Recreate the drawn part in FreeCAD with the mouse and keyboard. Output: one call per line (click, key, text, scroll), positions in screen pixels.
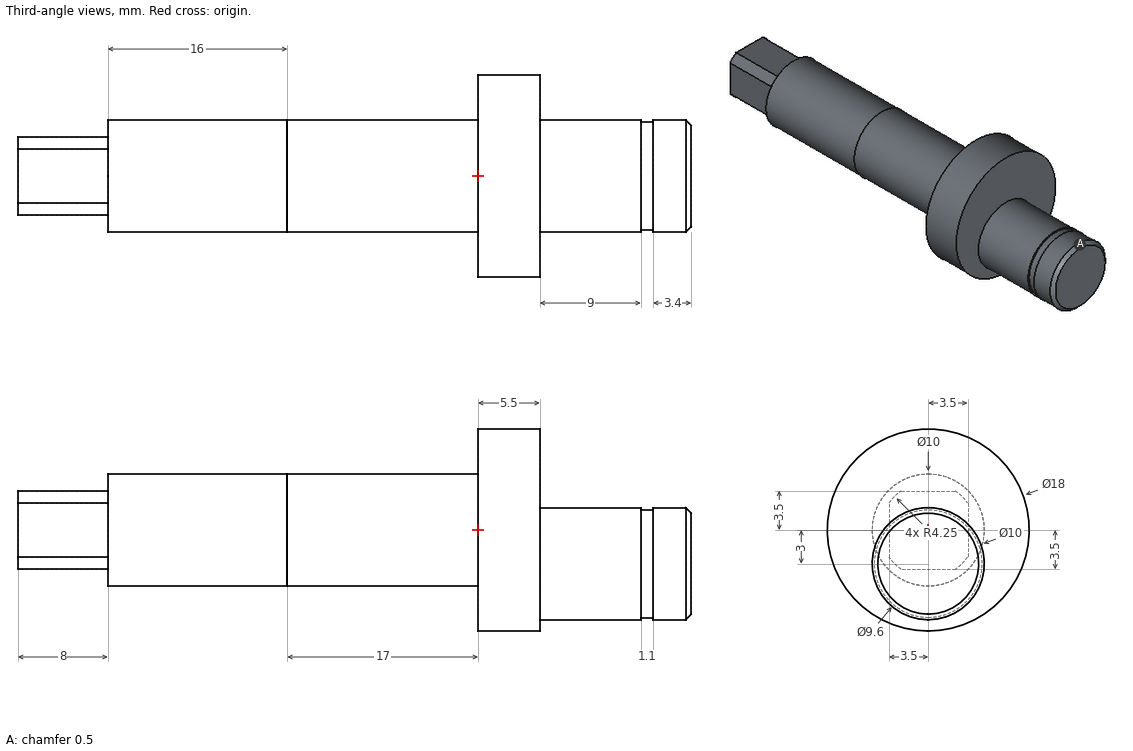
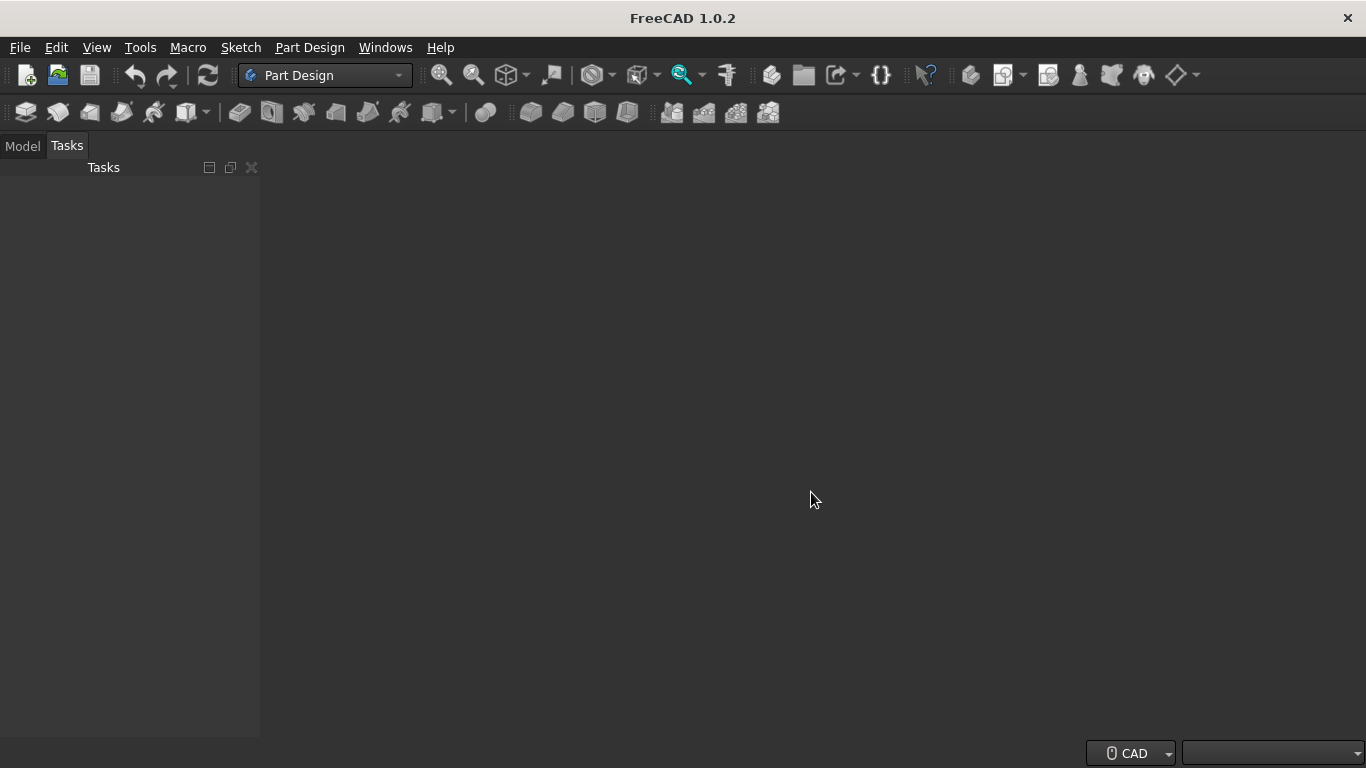
key(ctrl+n)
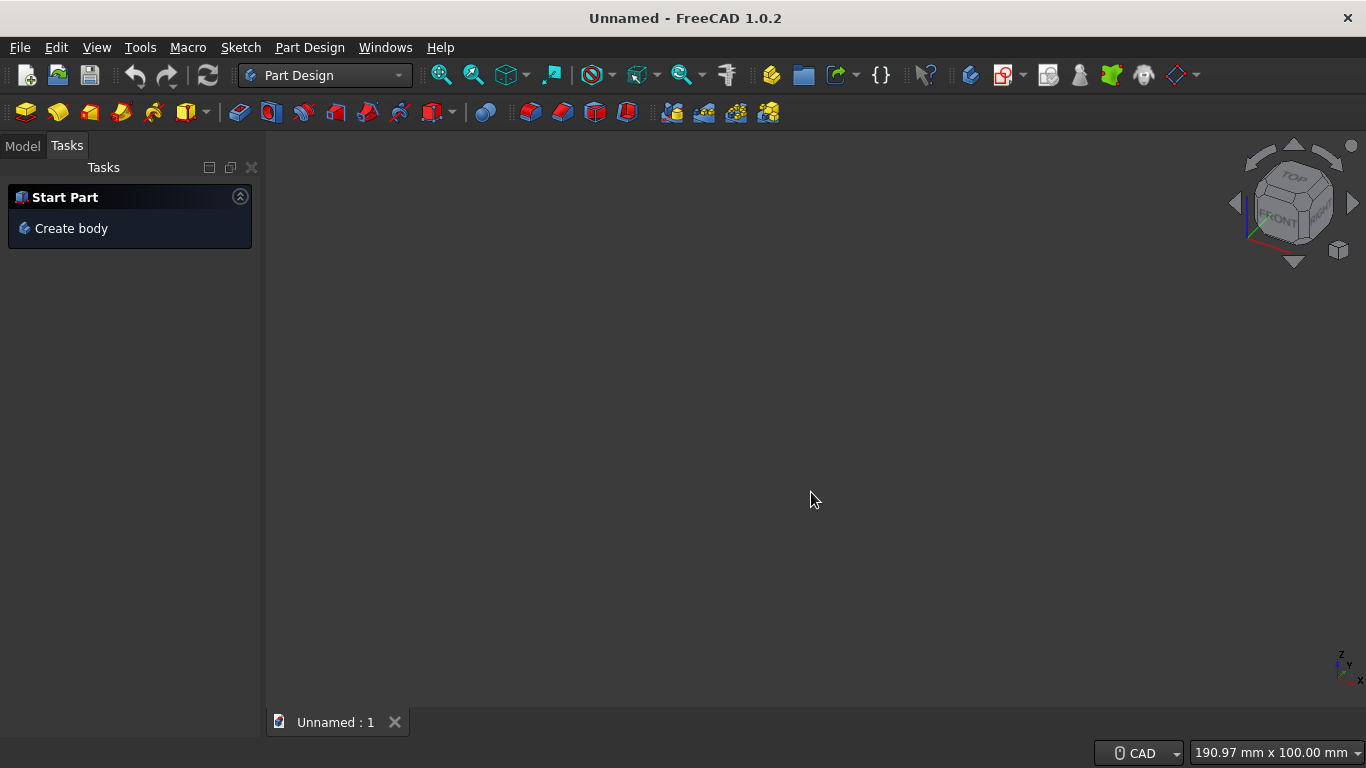
click(1004, 76)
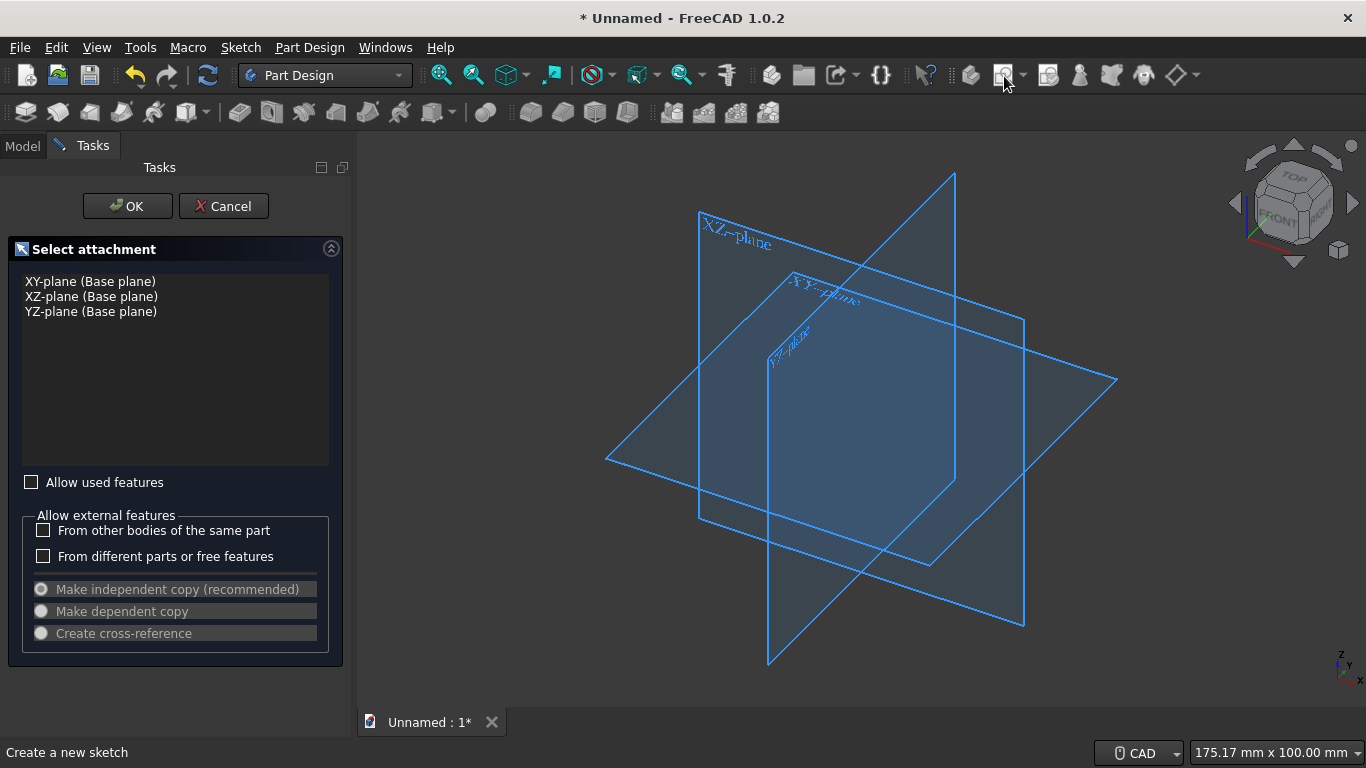
click(82, 312)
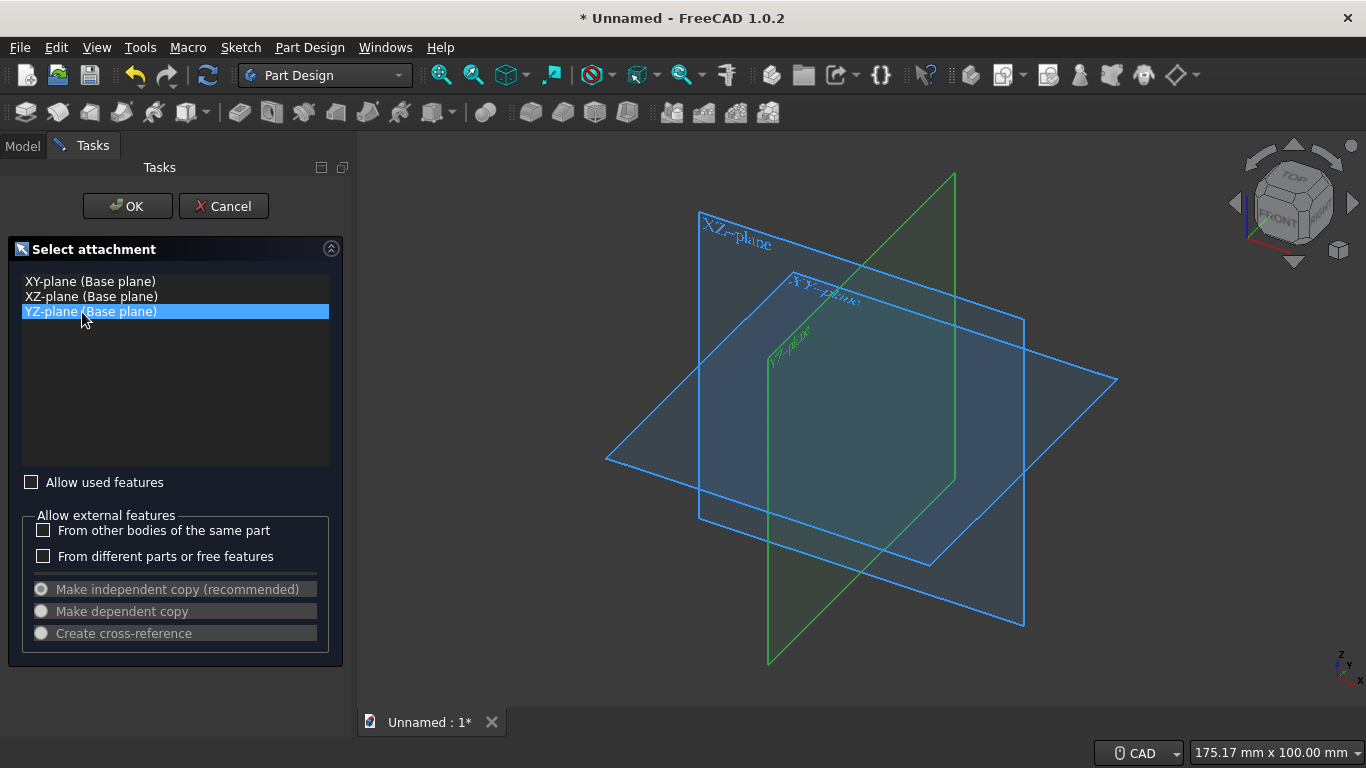
click(128, 206)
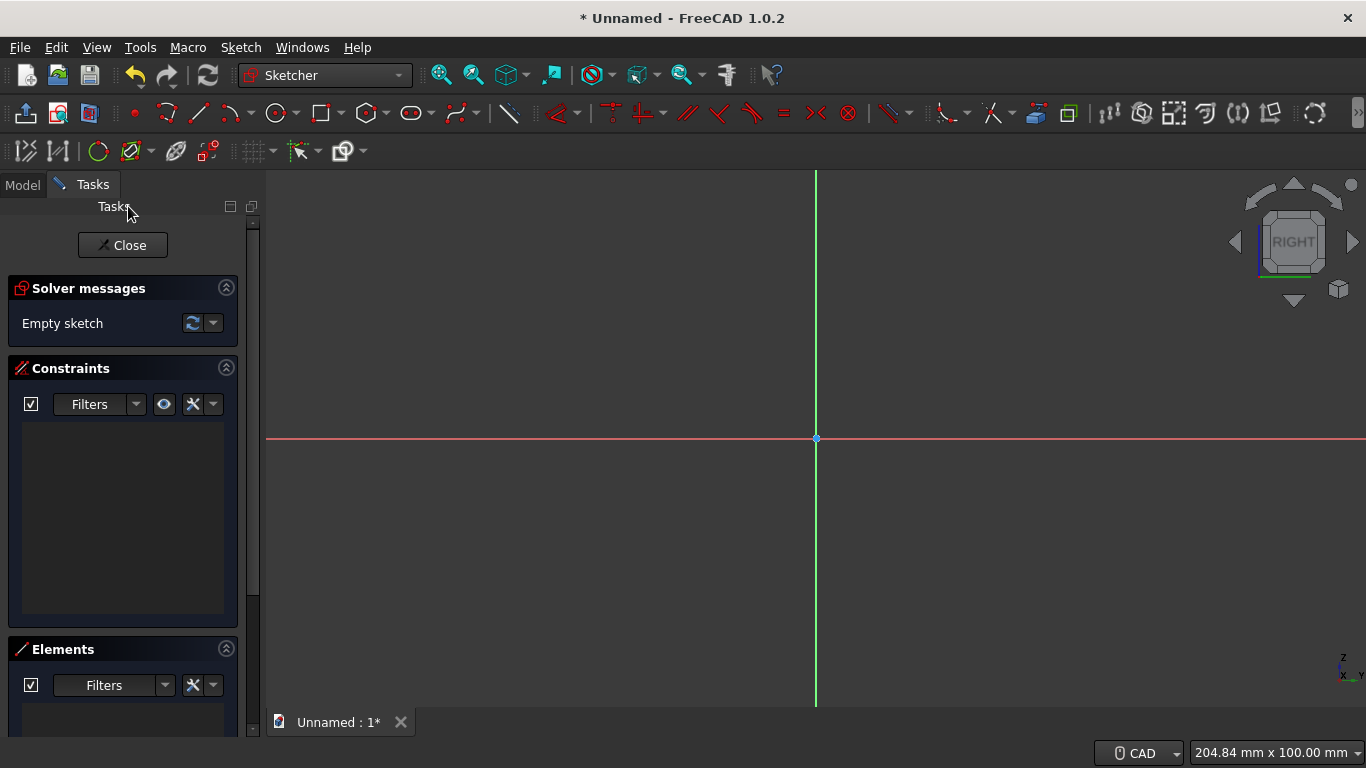
scroll(846, 438, up, 6)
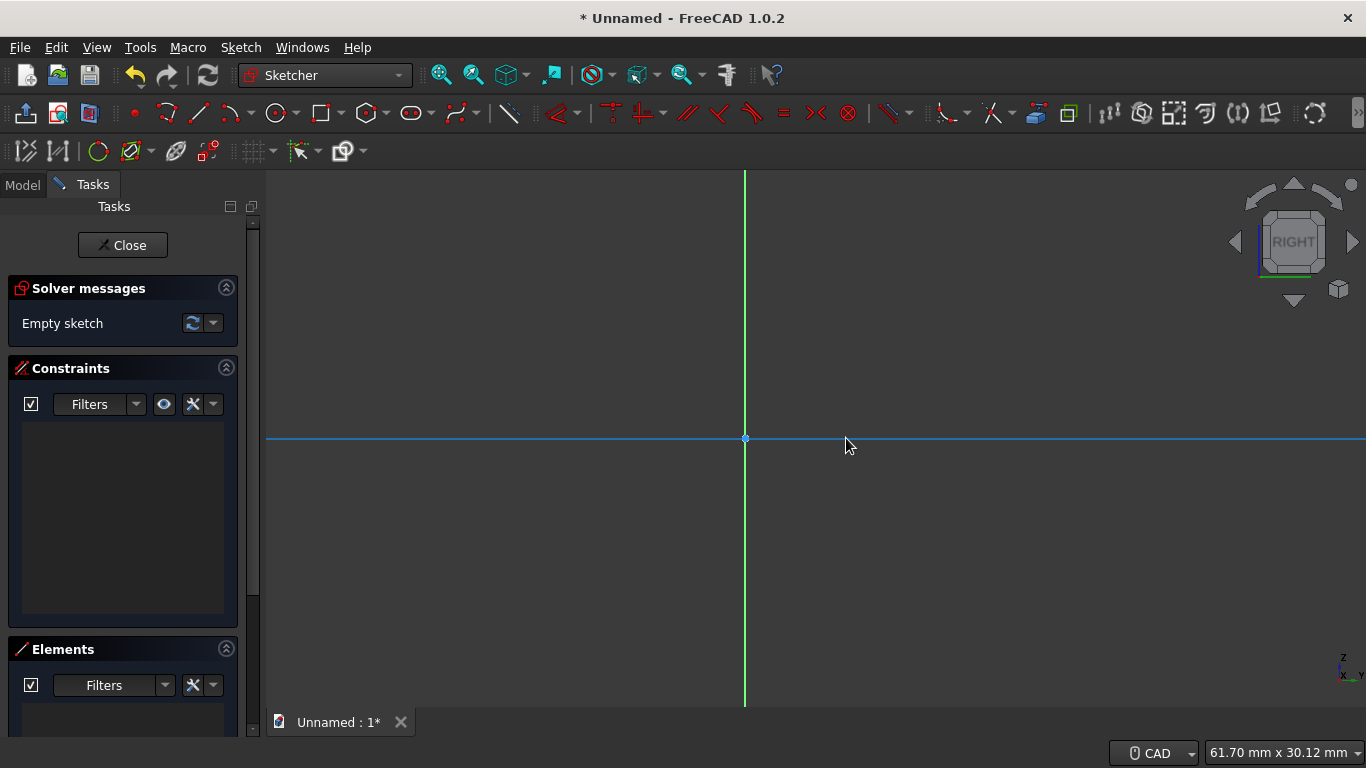
key(g)
key(c)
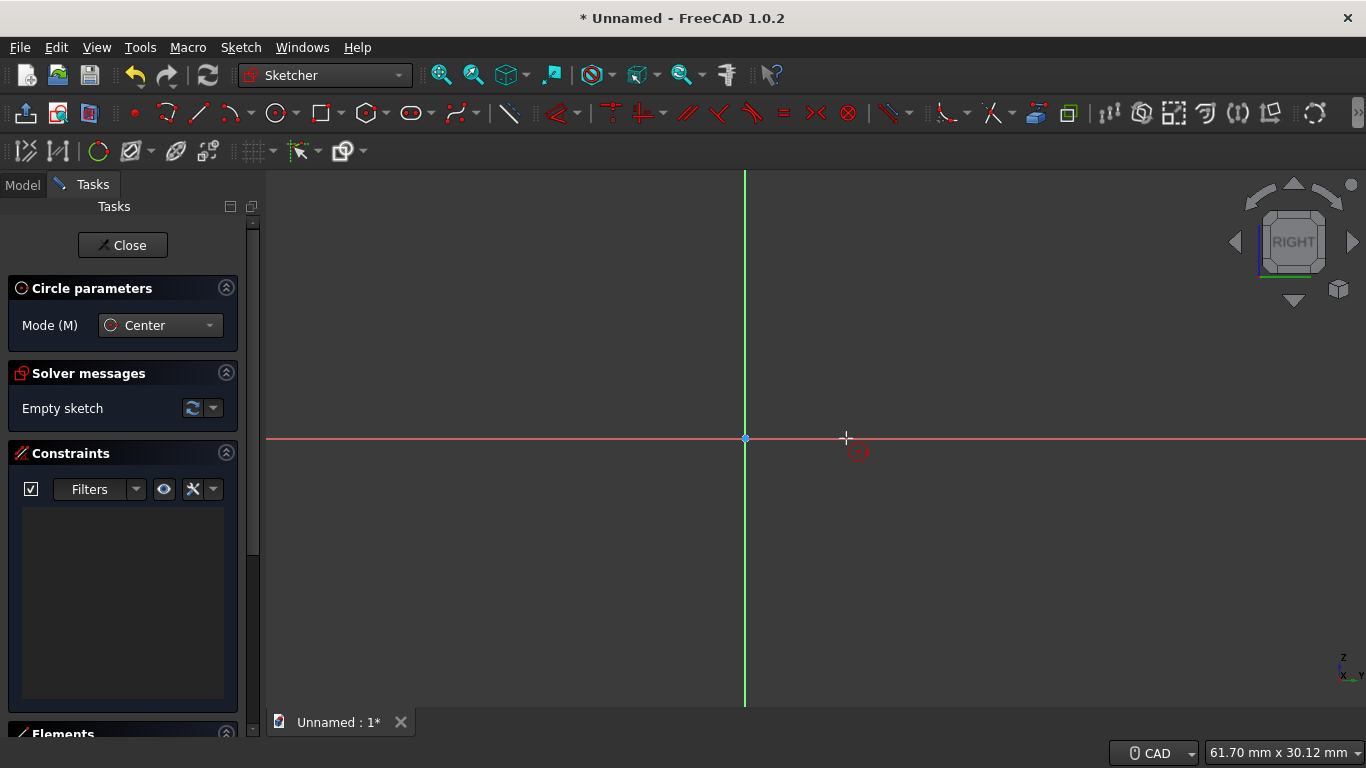
click(745, 438)
click(859, 325)
key(Escape)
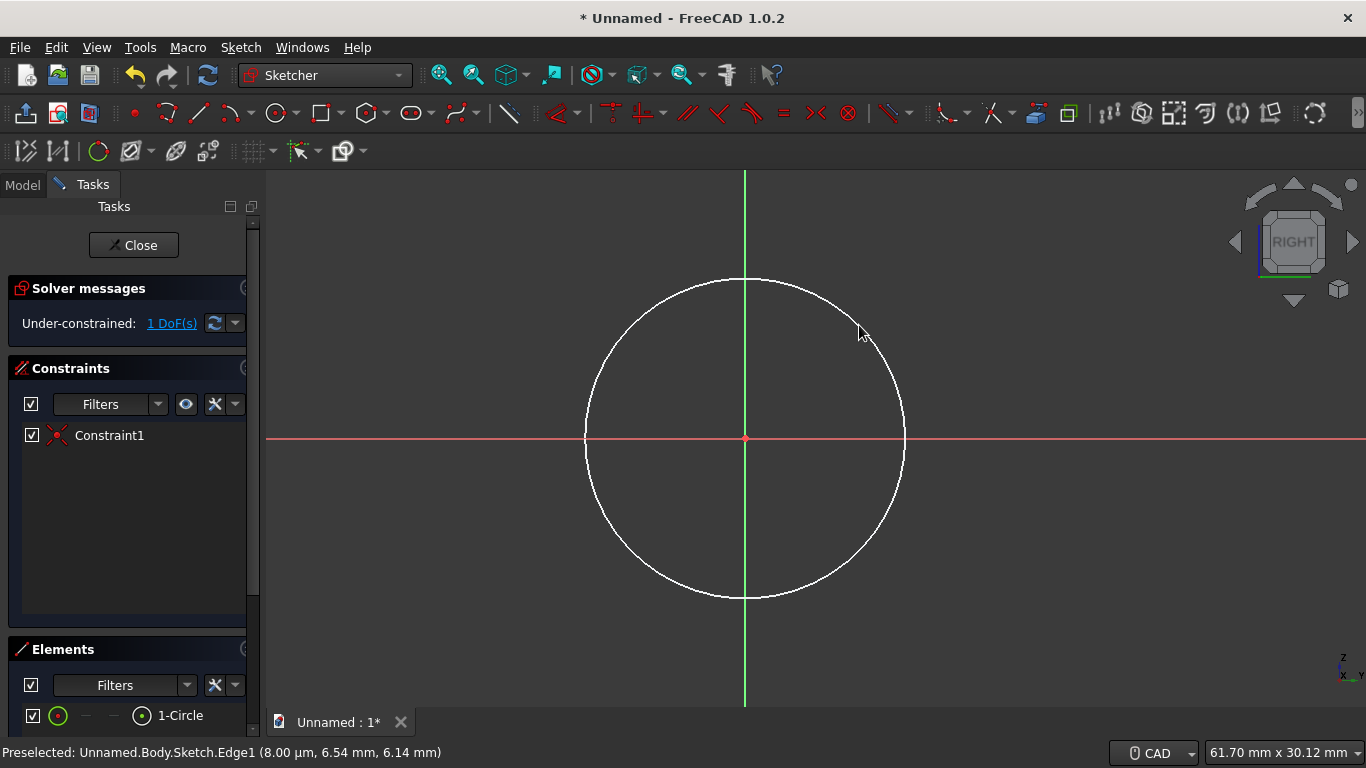
key(d)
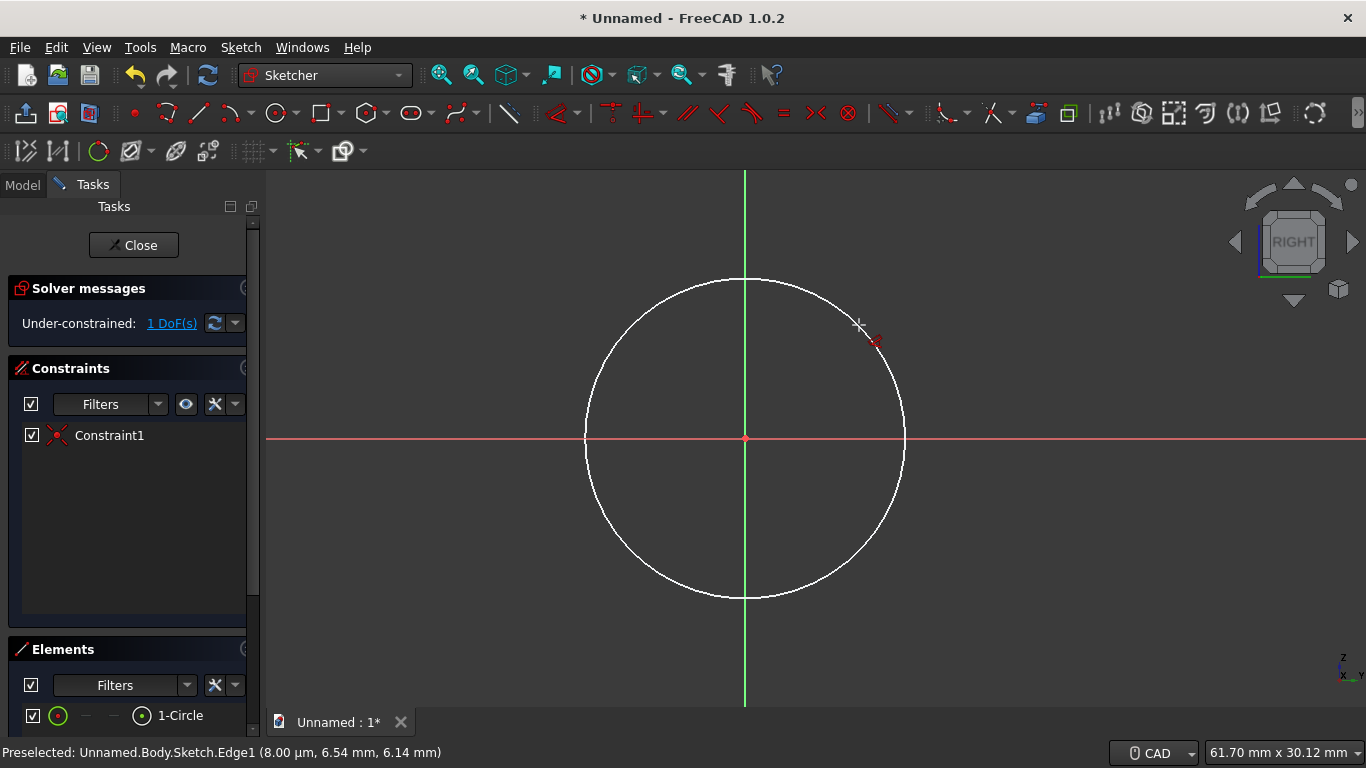
click(858, 325)
click(881, 302)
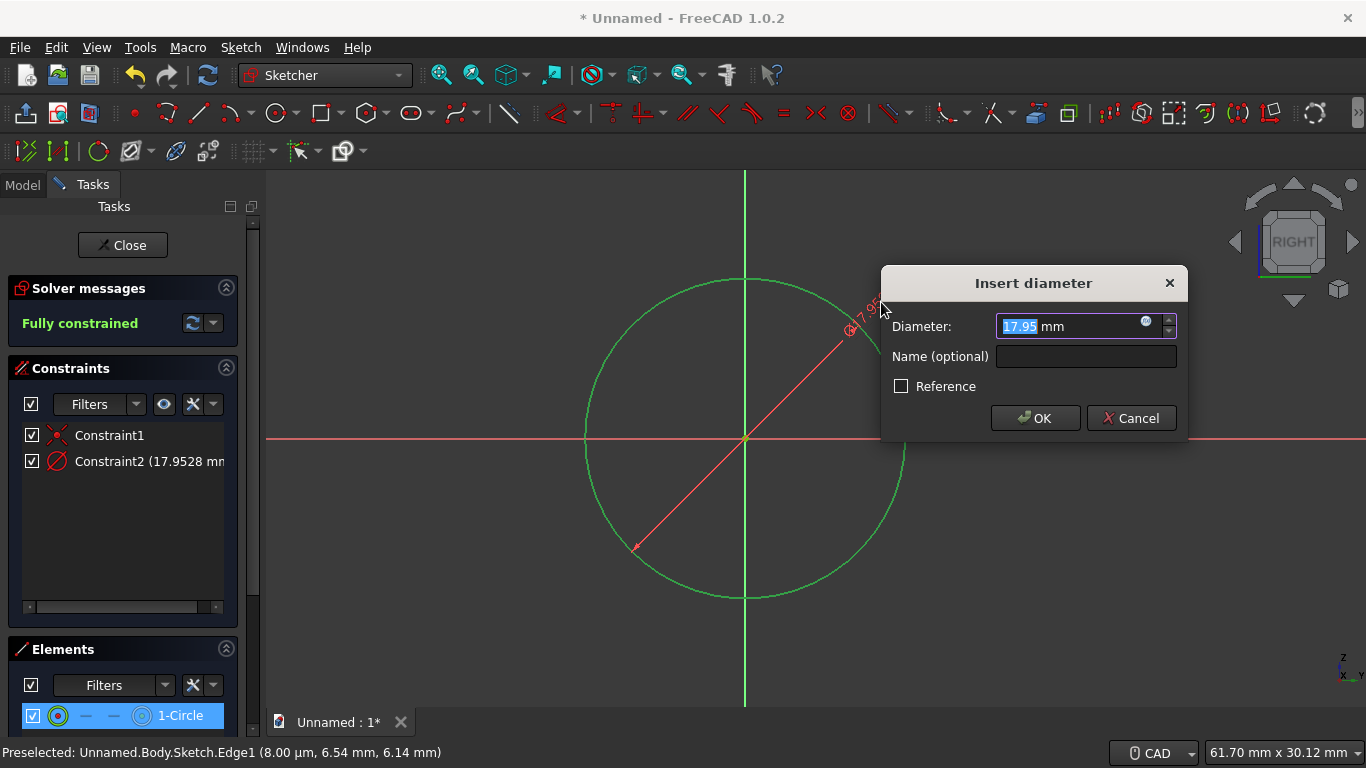
text(18)
key(Return)
key(Escape)